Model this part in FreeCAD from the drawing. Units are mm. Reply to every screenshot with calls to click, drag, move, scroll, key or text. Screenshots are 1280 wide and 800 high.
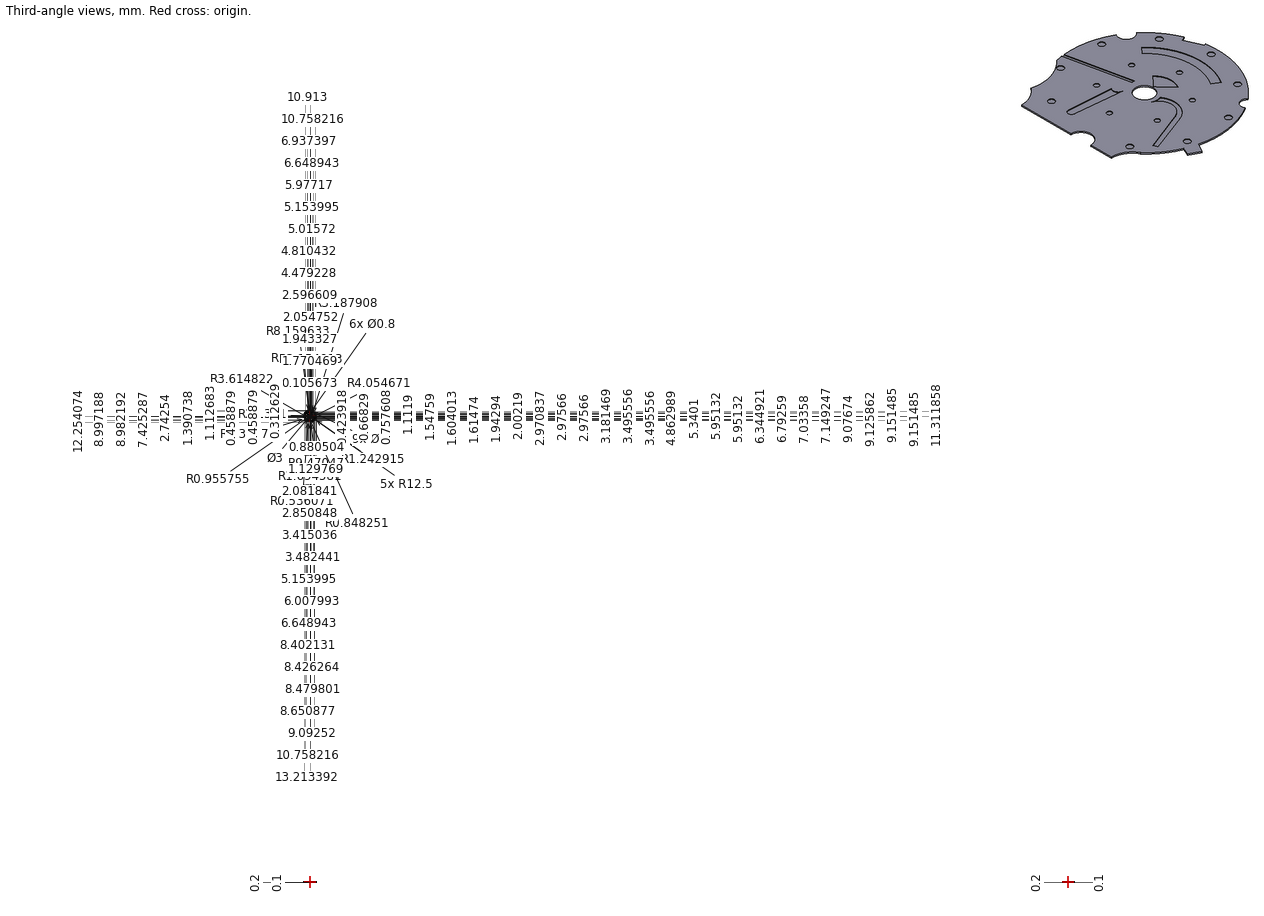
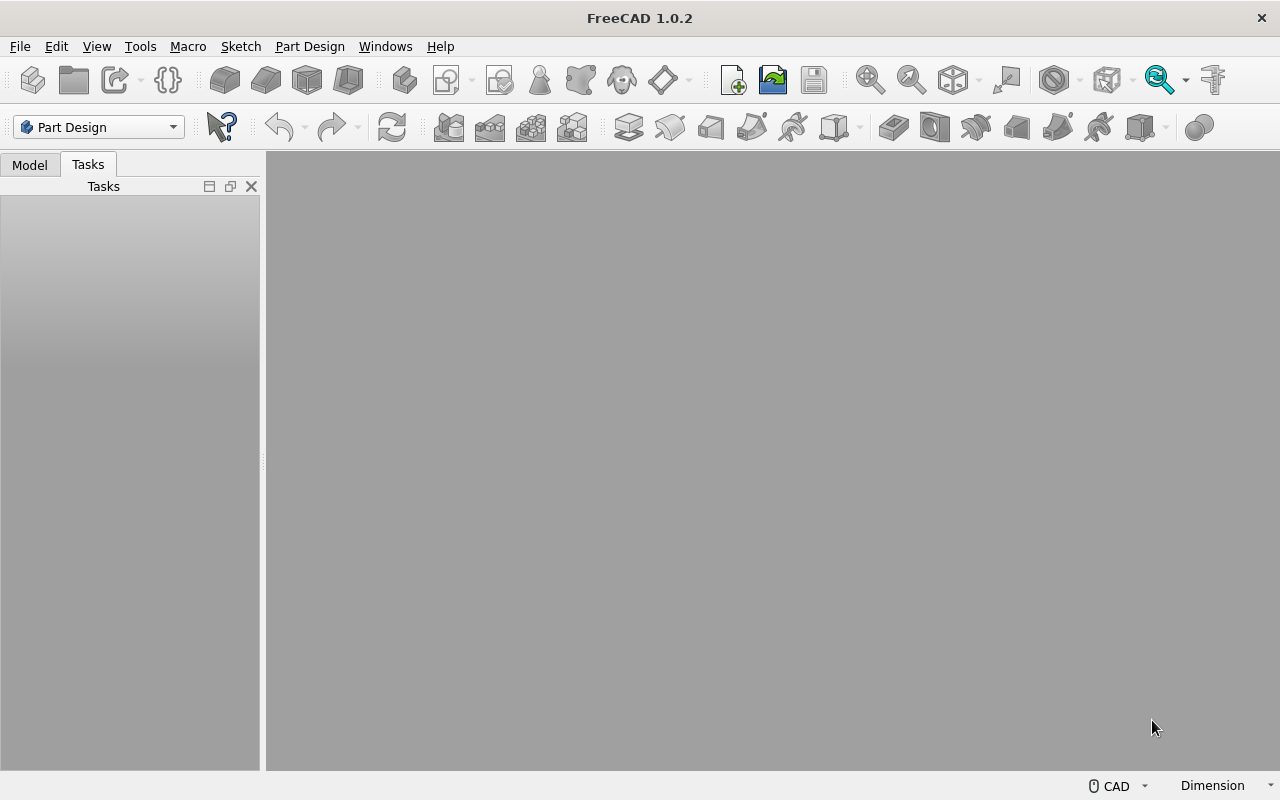
click(732, 80)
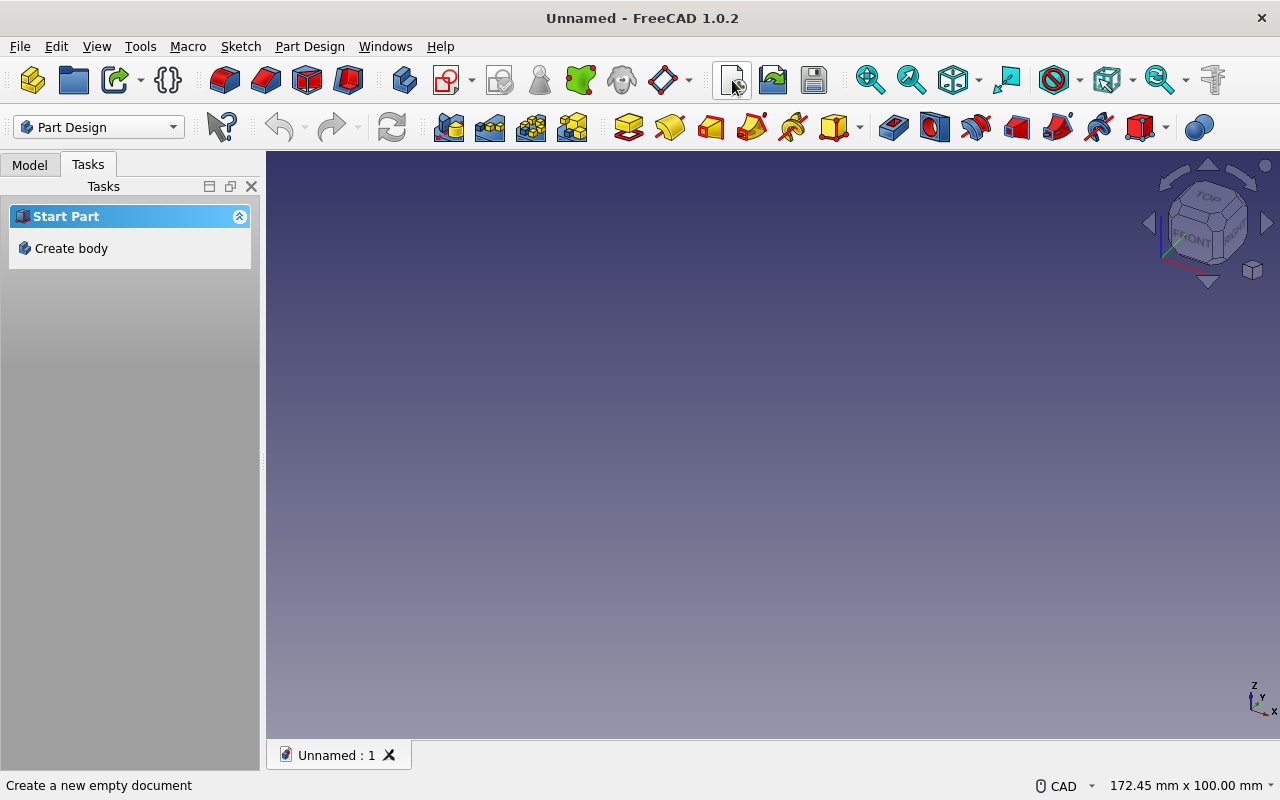
click(446, 80)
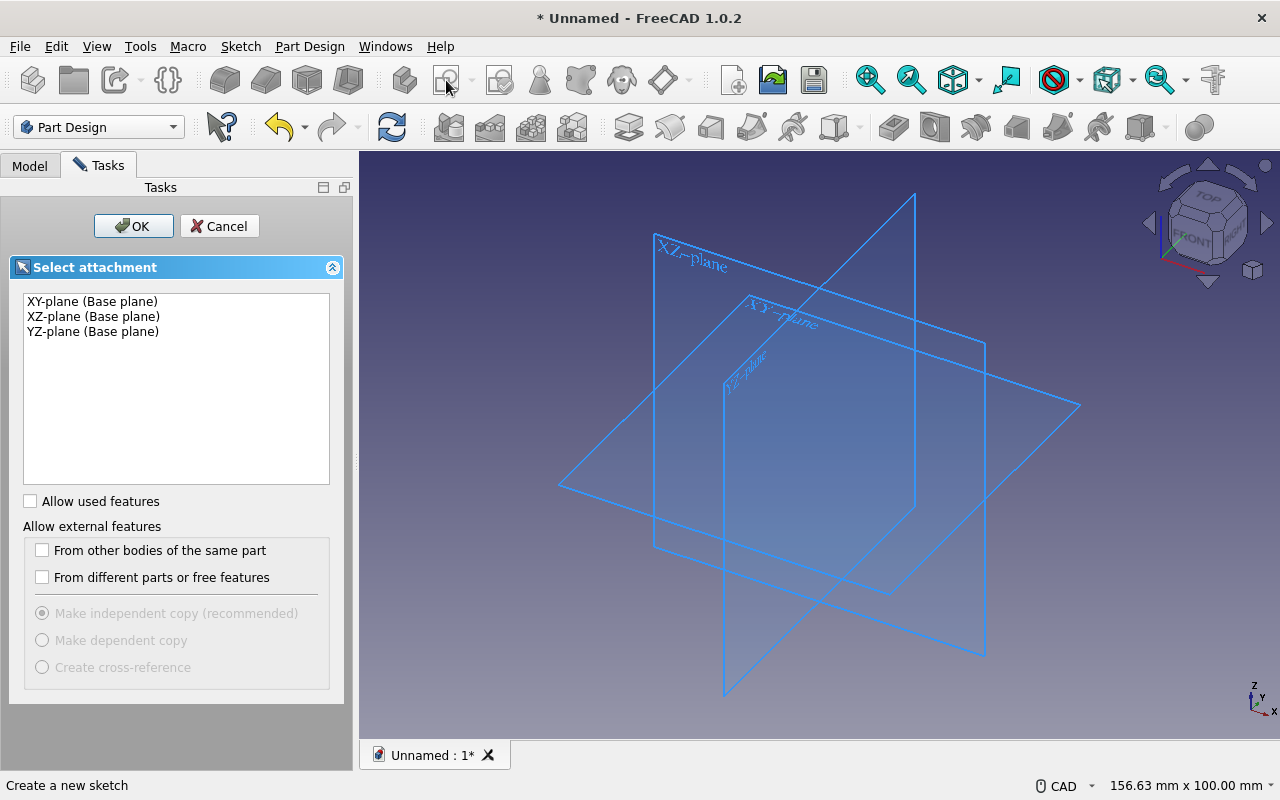
click(84, 302)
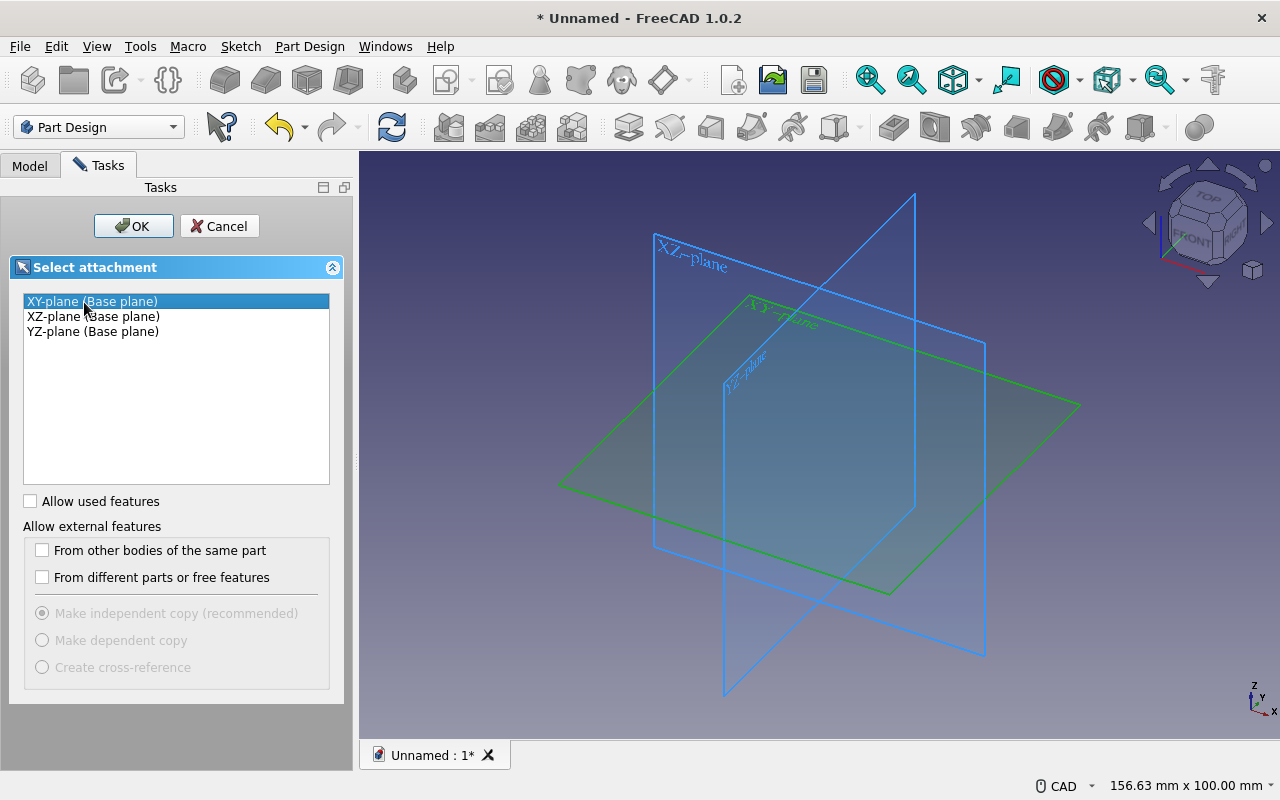
click(134, 226)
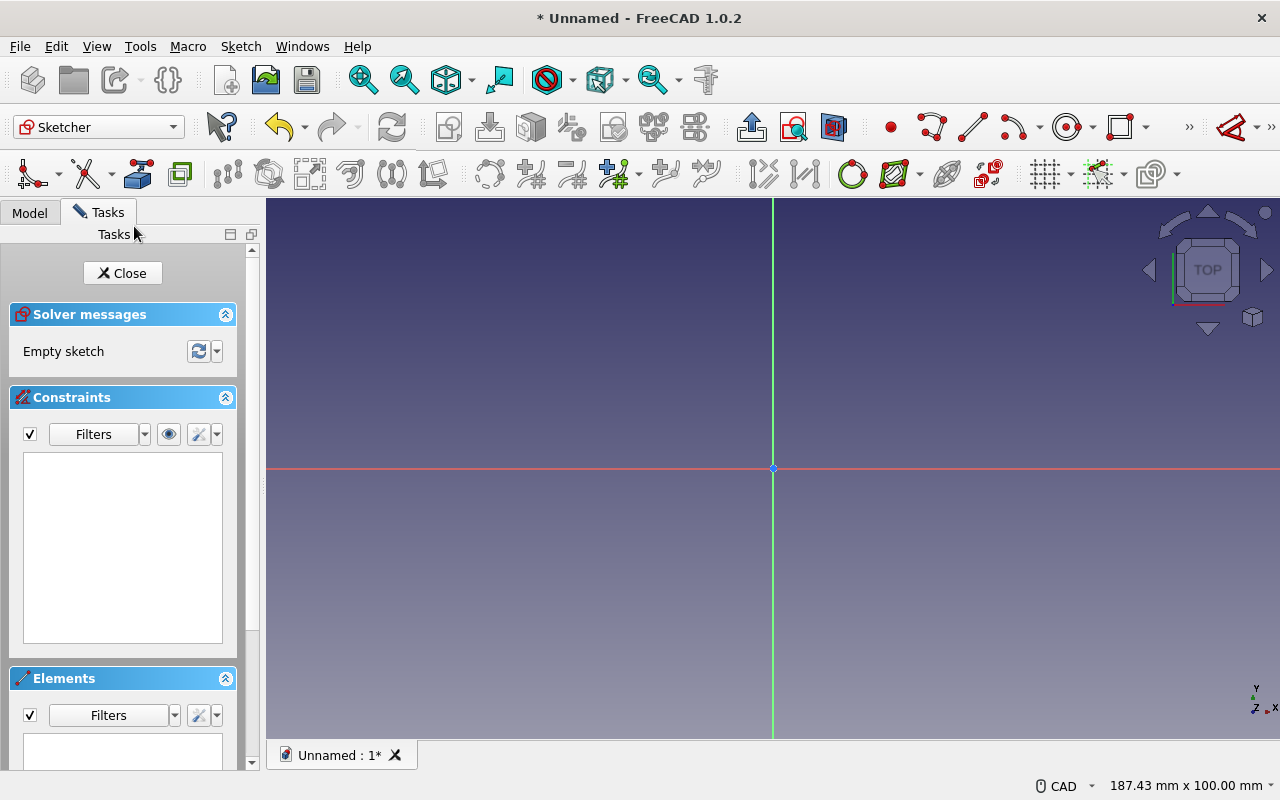
scroll(818, 468, up, 5)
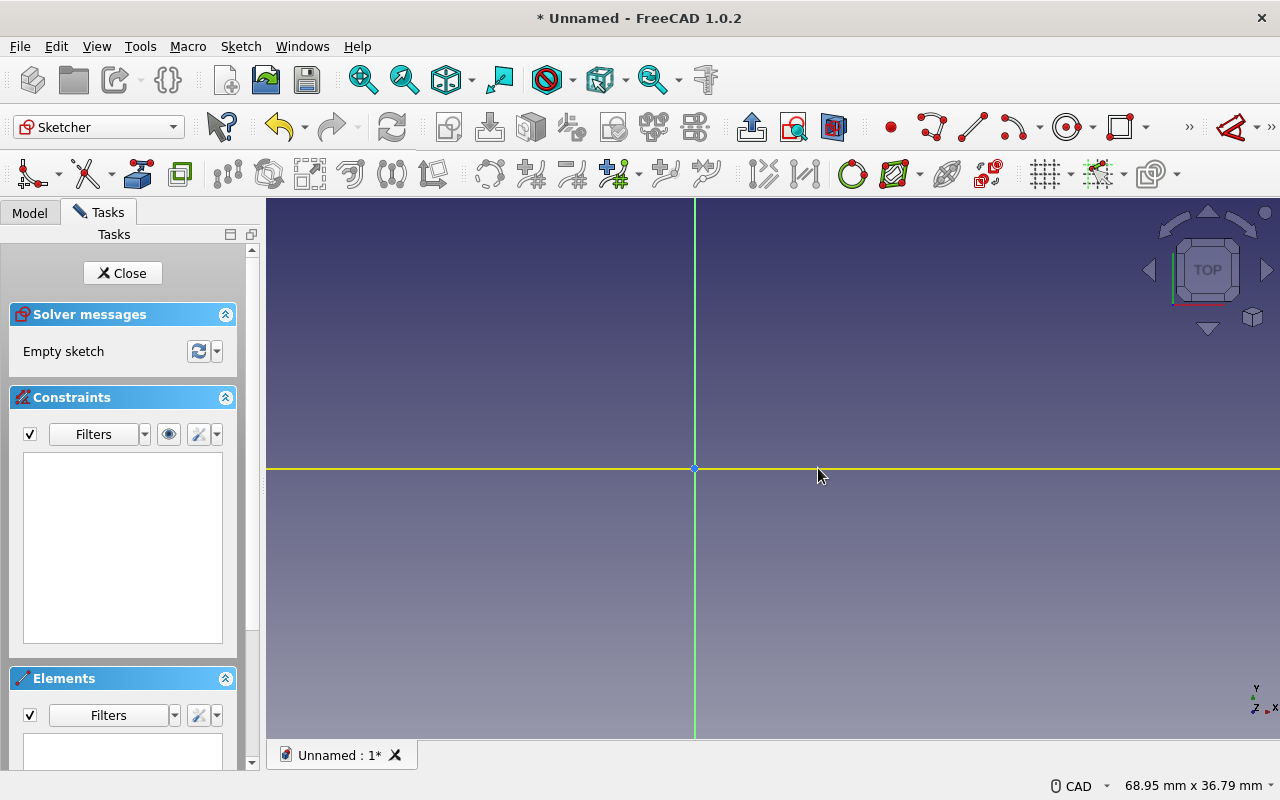
key(g)
key(l)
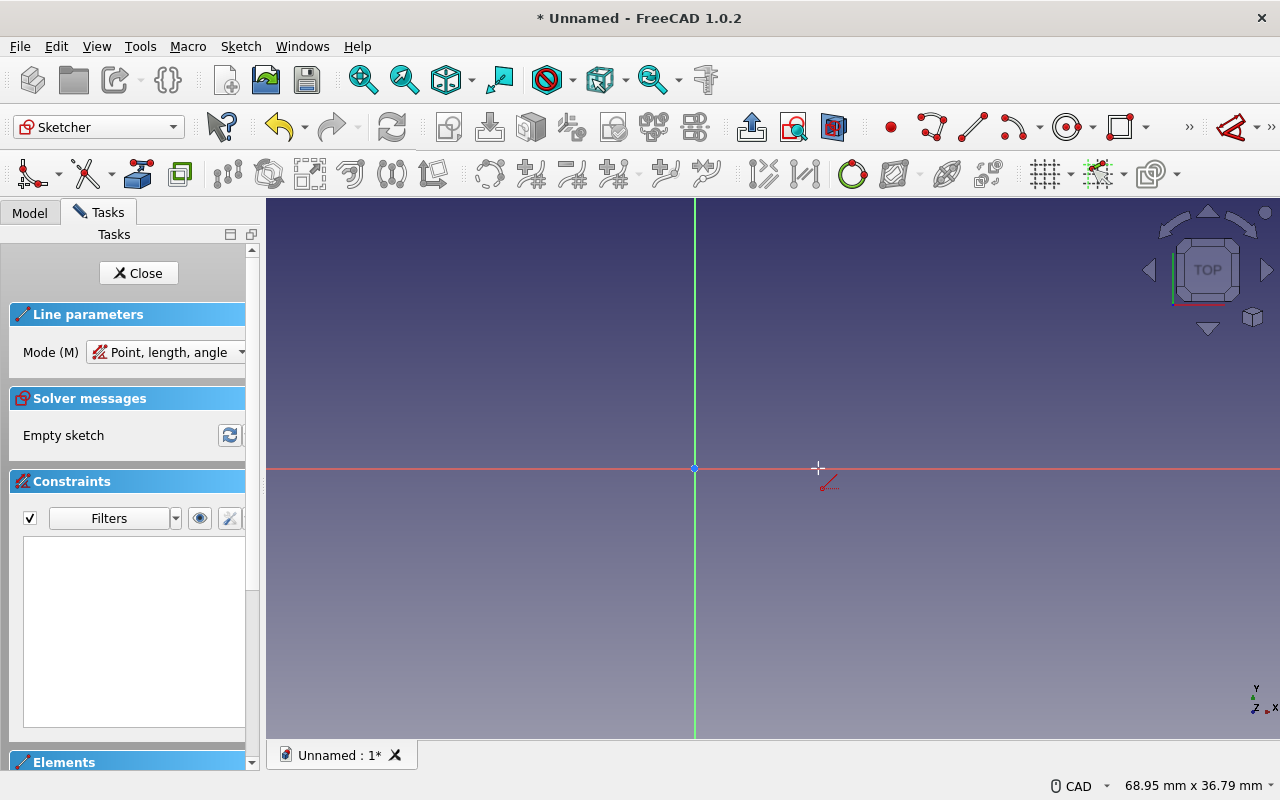
click(568, 649)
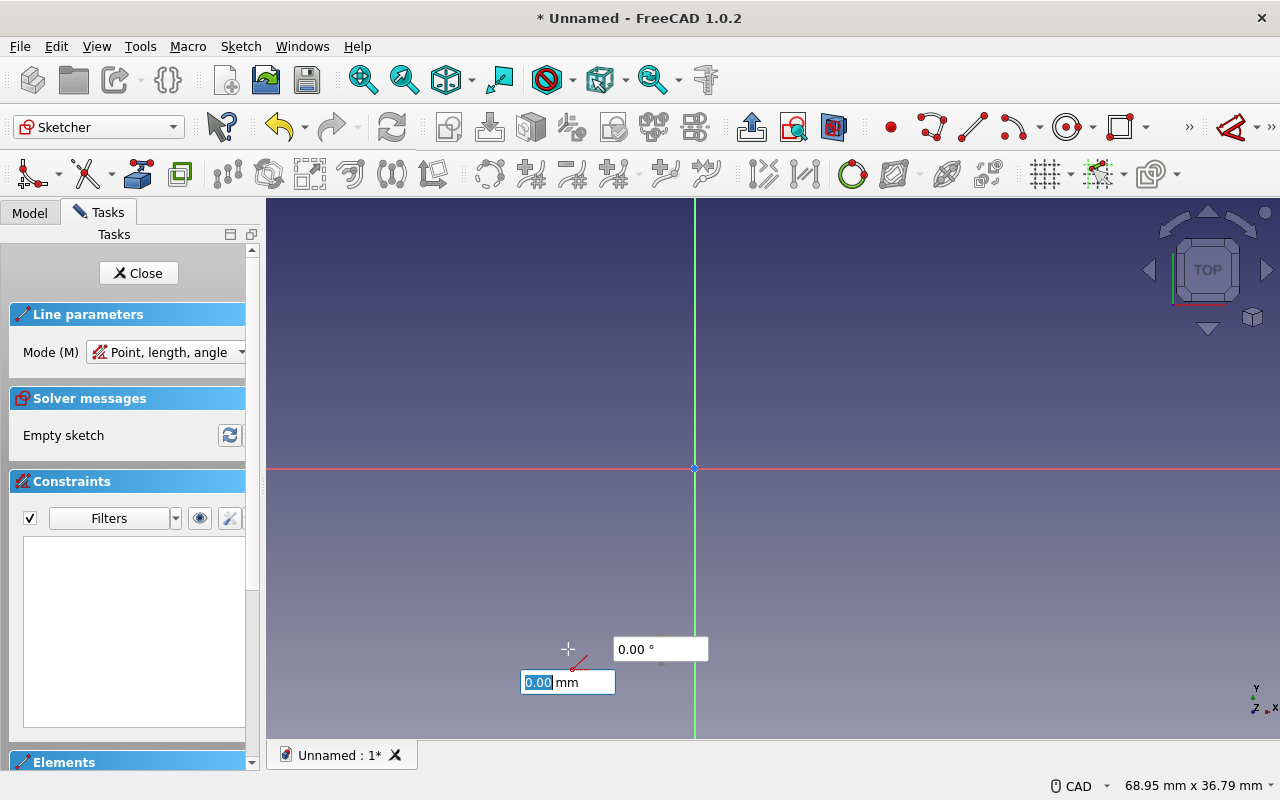
scroll(691, 649, up, 8)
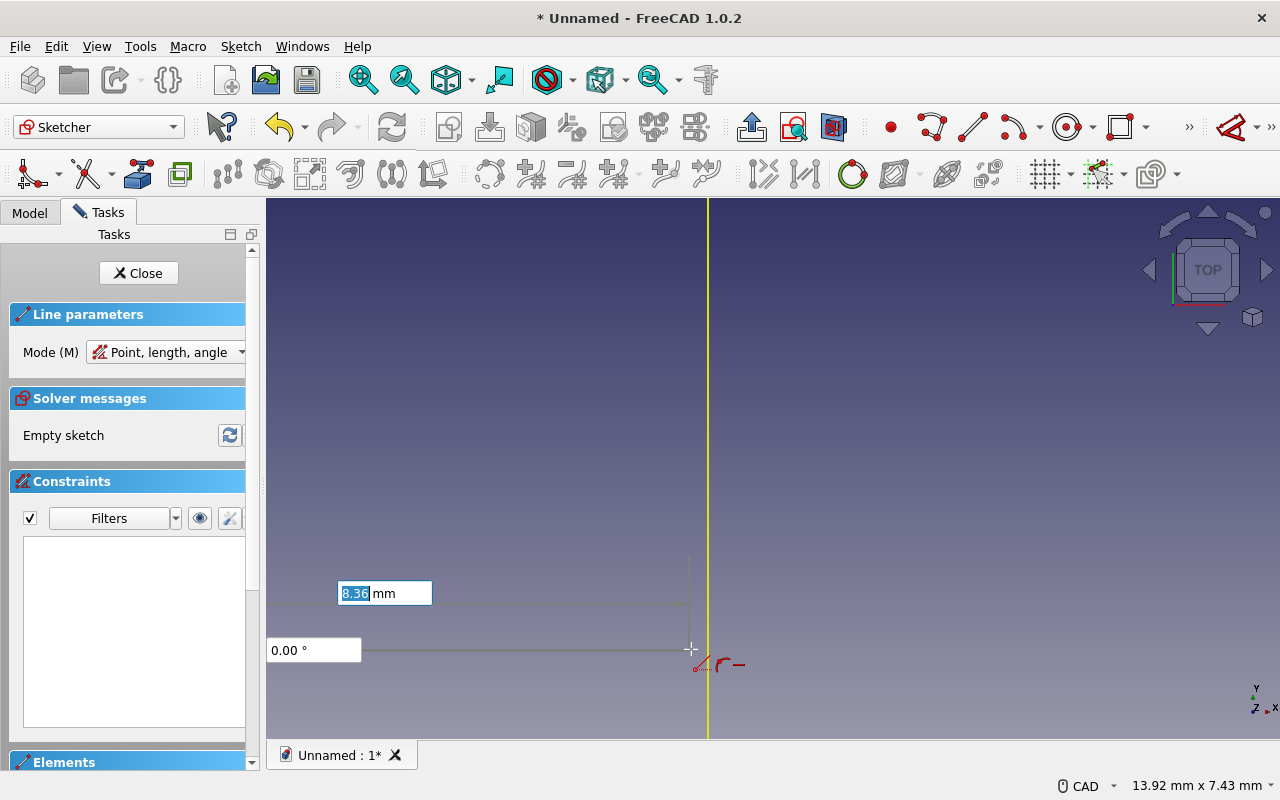
click(690, 646)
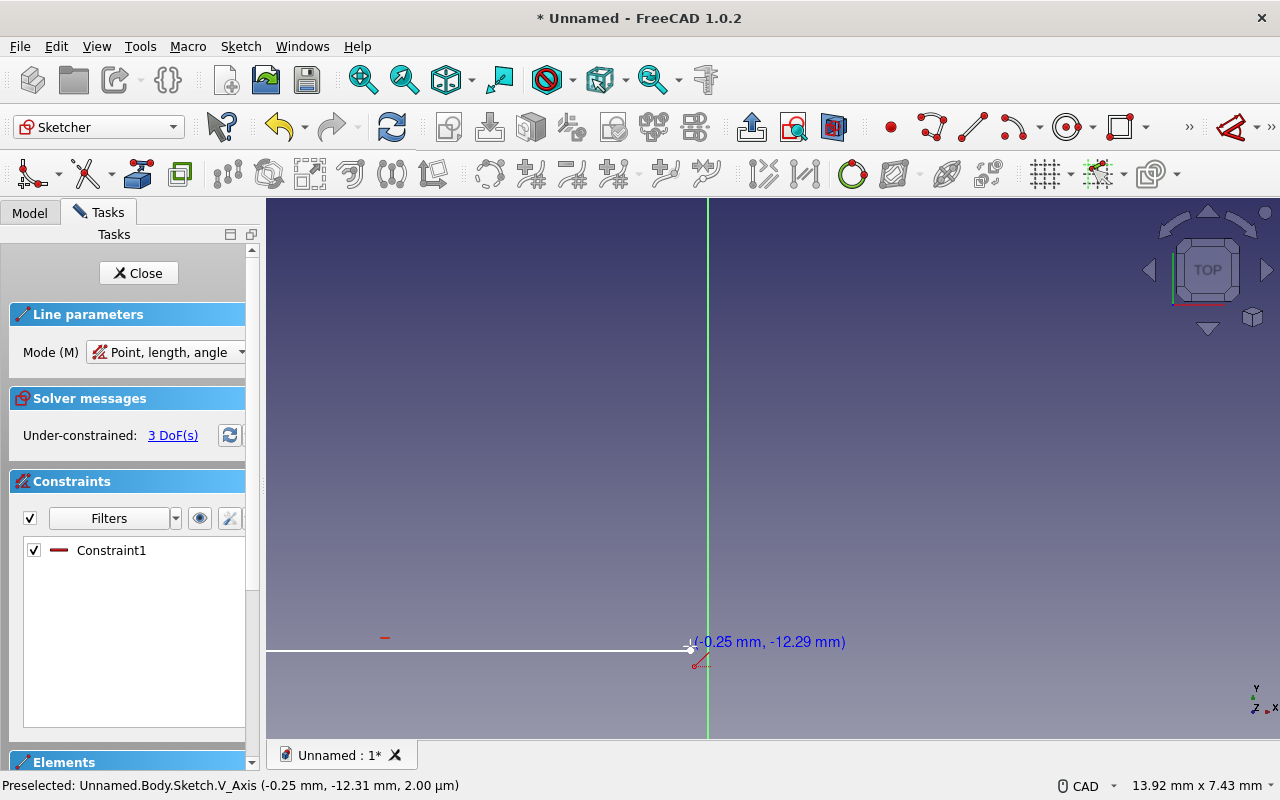
scroll(693, 651, down, 8)